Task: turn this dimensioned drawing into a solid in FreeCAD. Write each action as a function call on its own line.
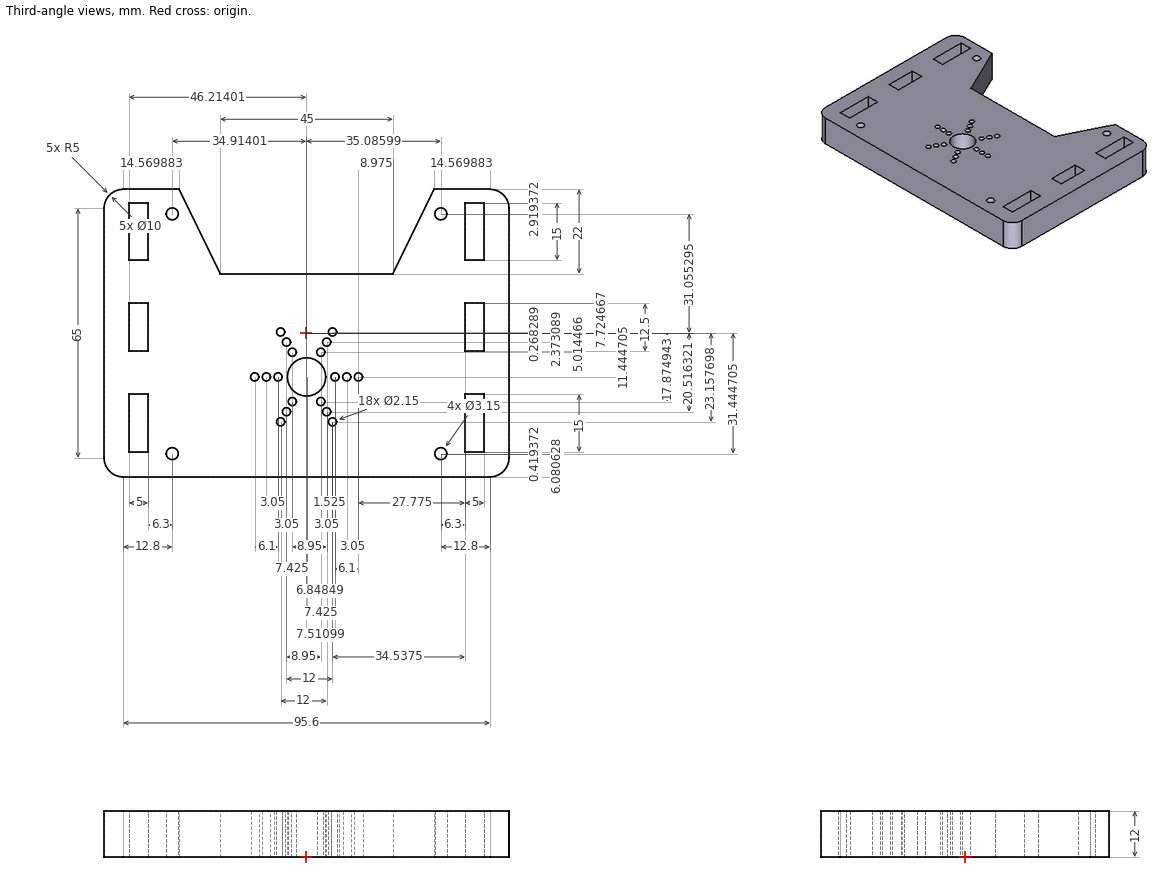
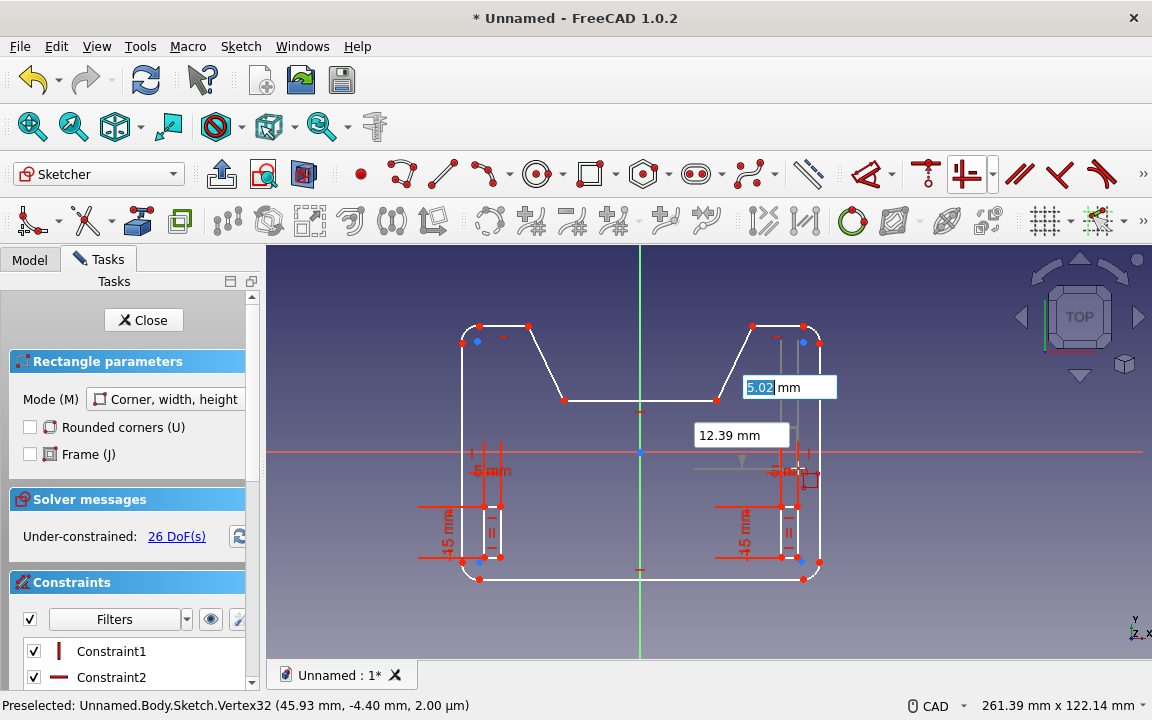
text(5)
key(Tab)
text(12.5)
key(Return)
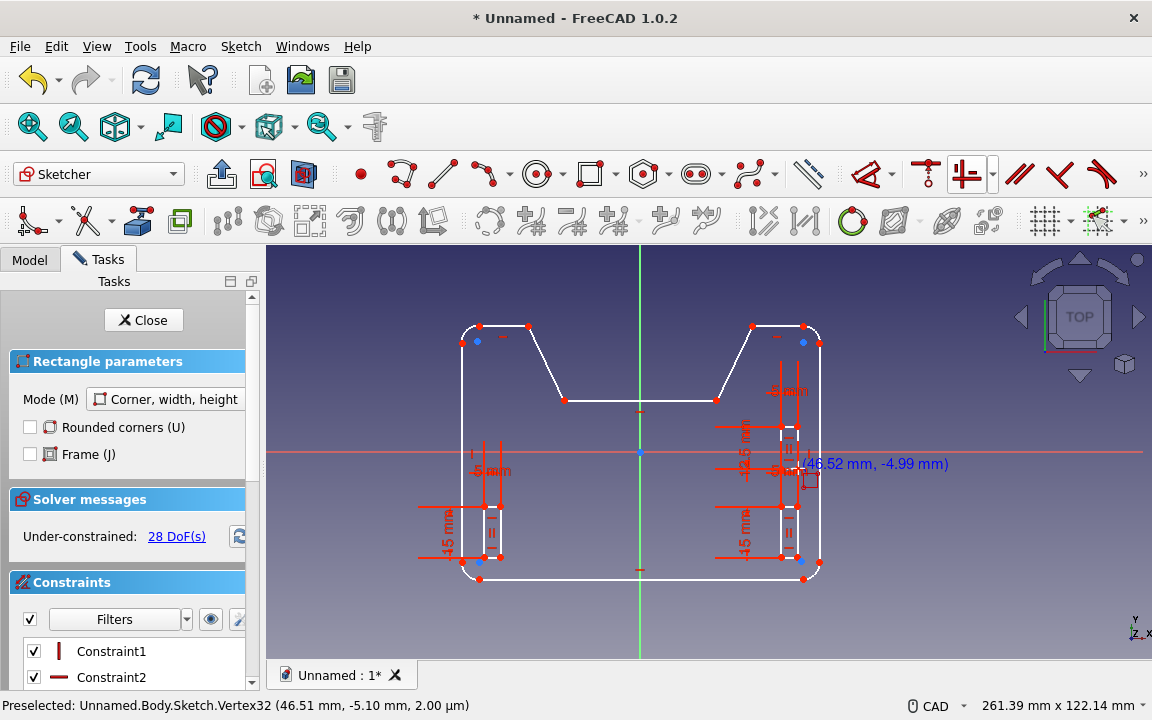
scroll(781, 337, up, 2)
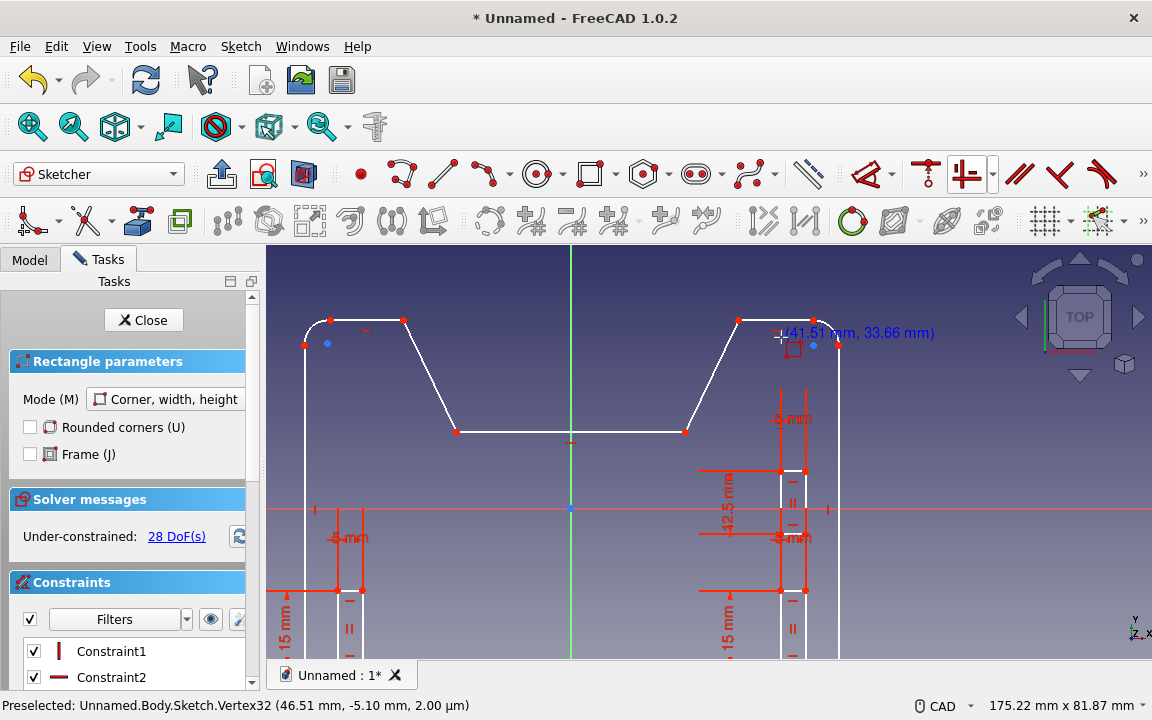
click(780, 337)
move(805, 413)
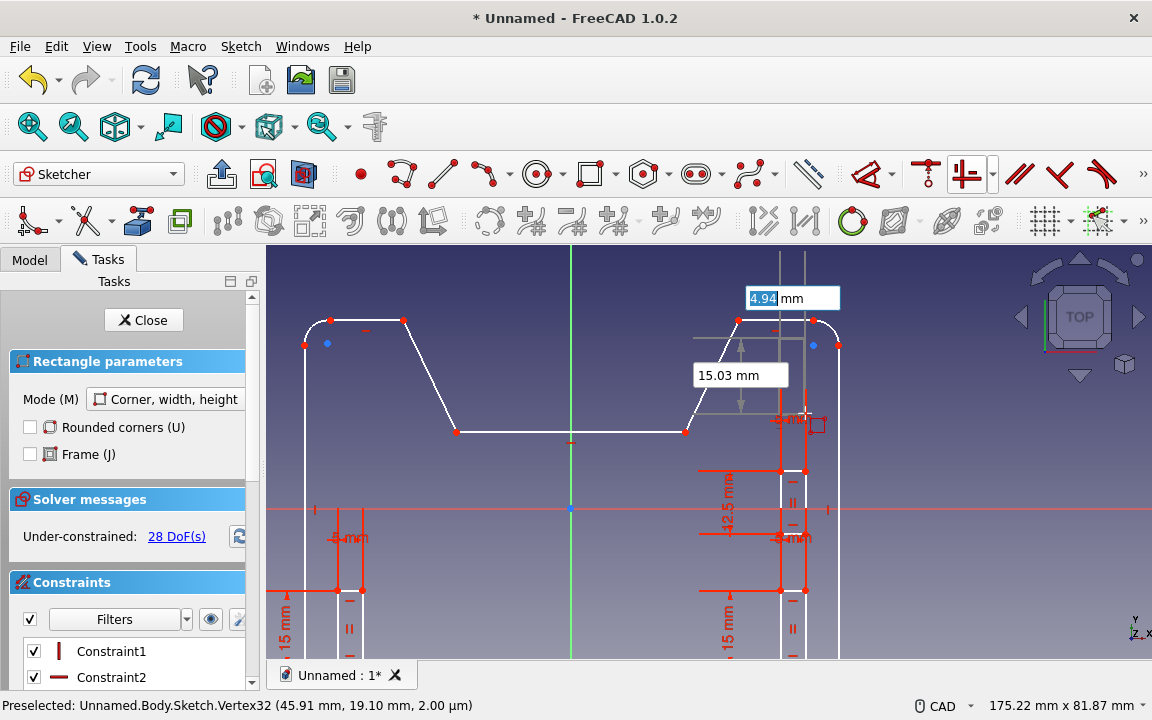
text(5)
key(Tab)
text(15)
key(Return)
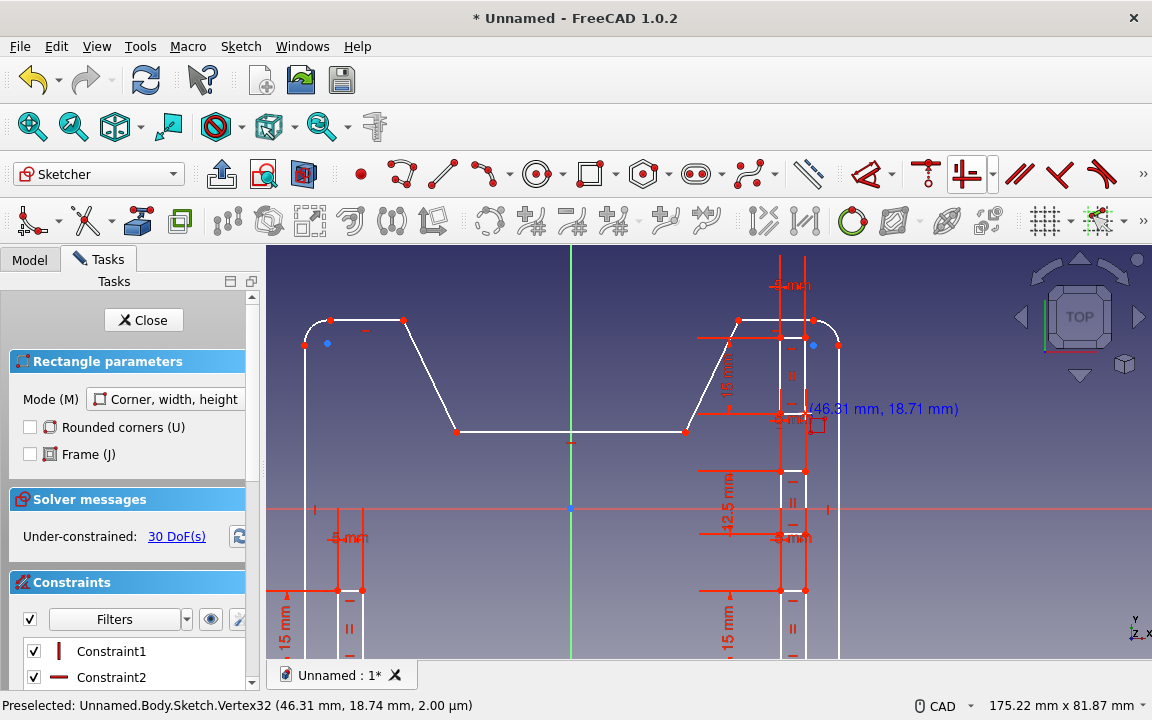
click(337, 470)
move(362, 533)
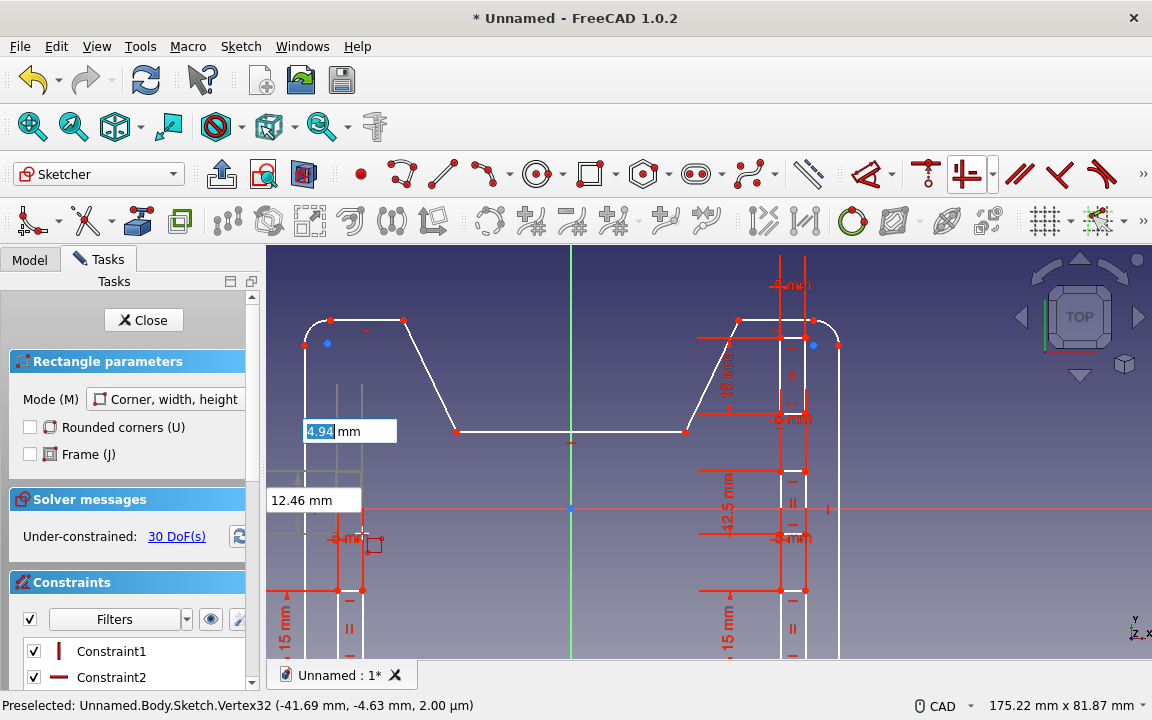
text(5)
key(Tab)
text(12.5)
key(Return)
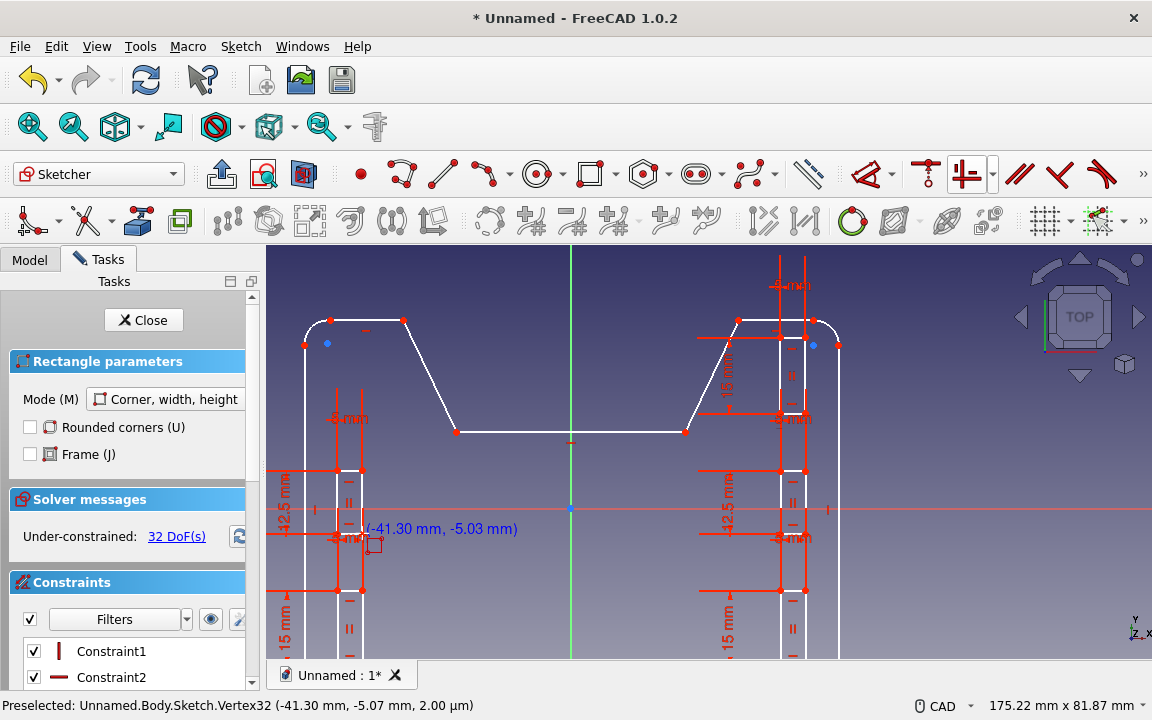
scroll(337, 337, up, 2)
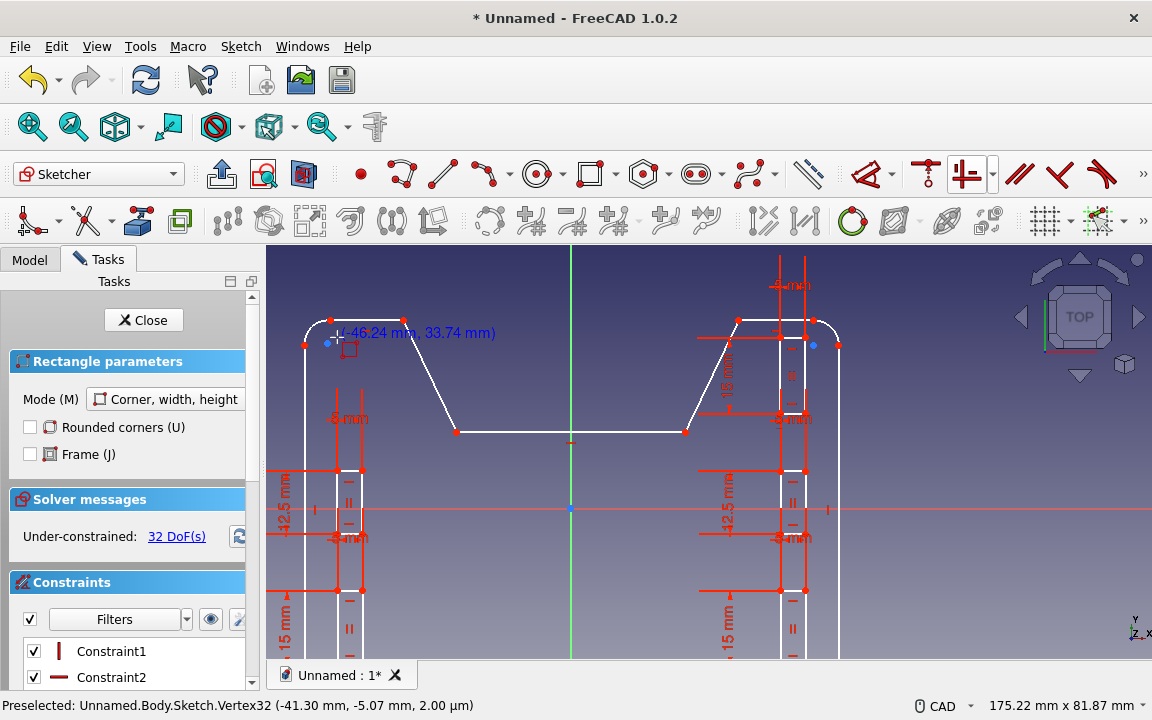
click(337, 337)
move(375, 450)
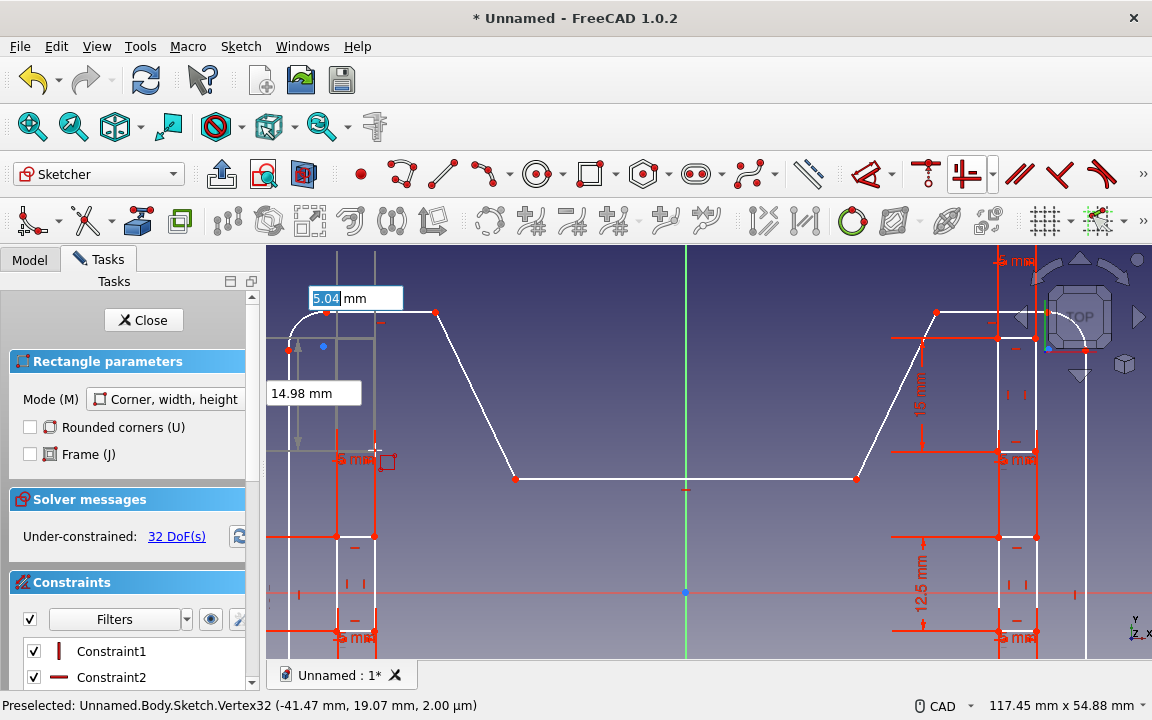
text(5)
key(Tab)
text(15)
key(Return)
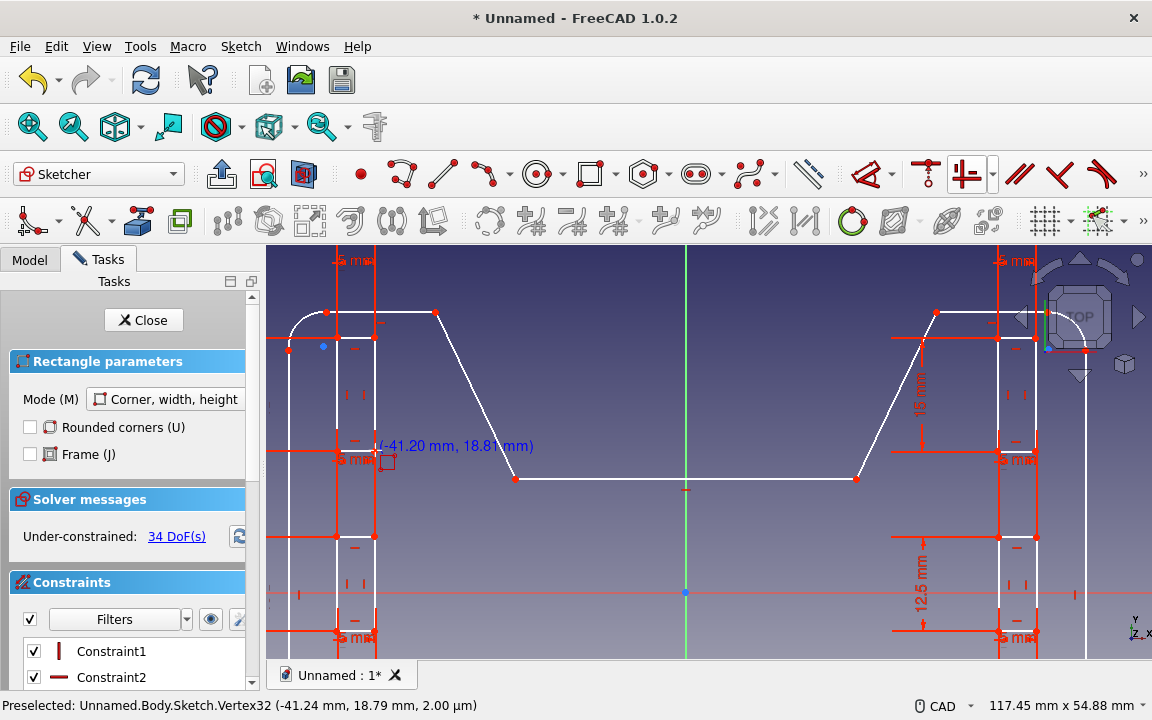
click(536, 174)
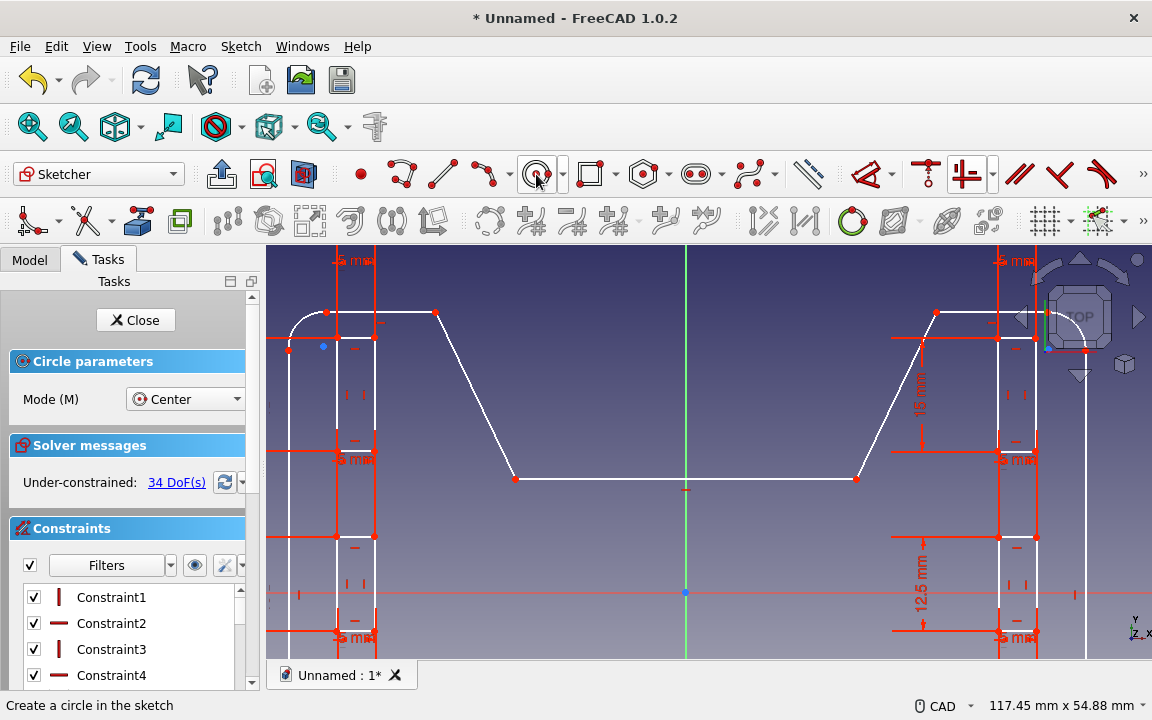
scroll(603, 337, down, 4)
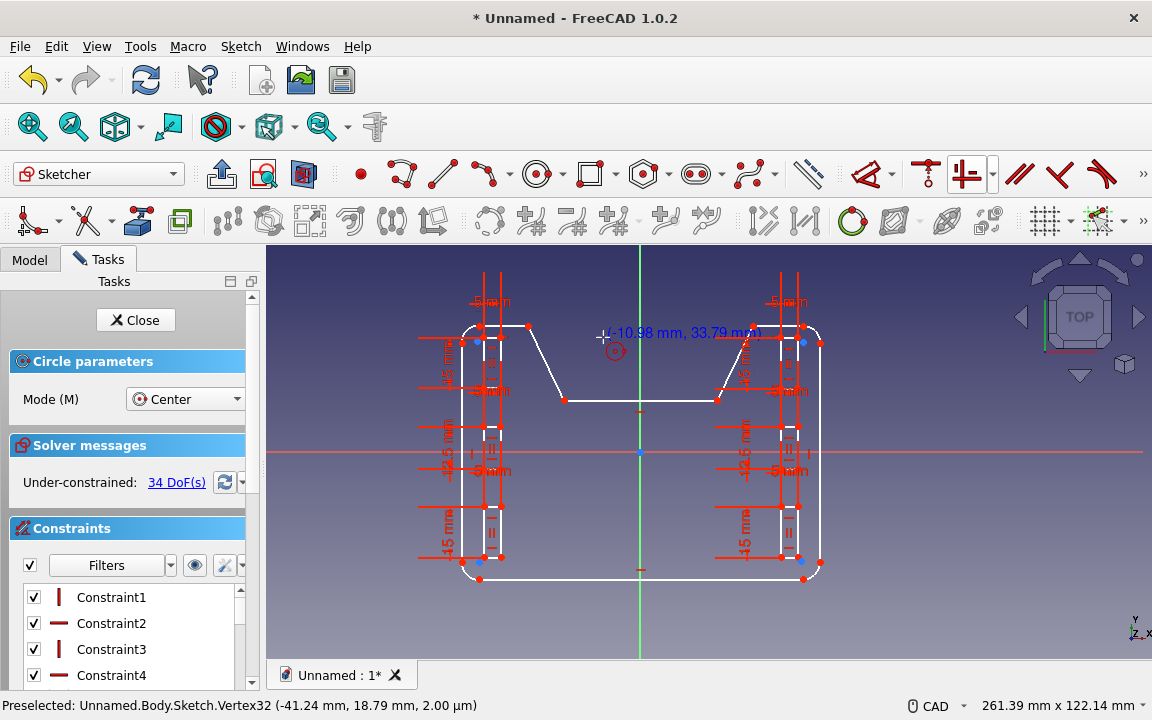
scroll(759, 559, up, 8)